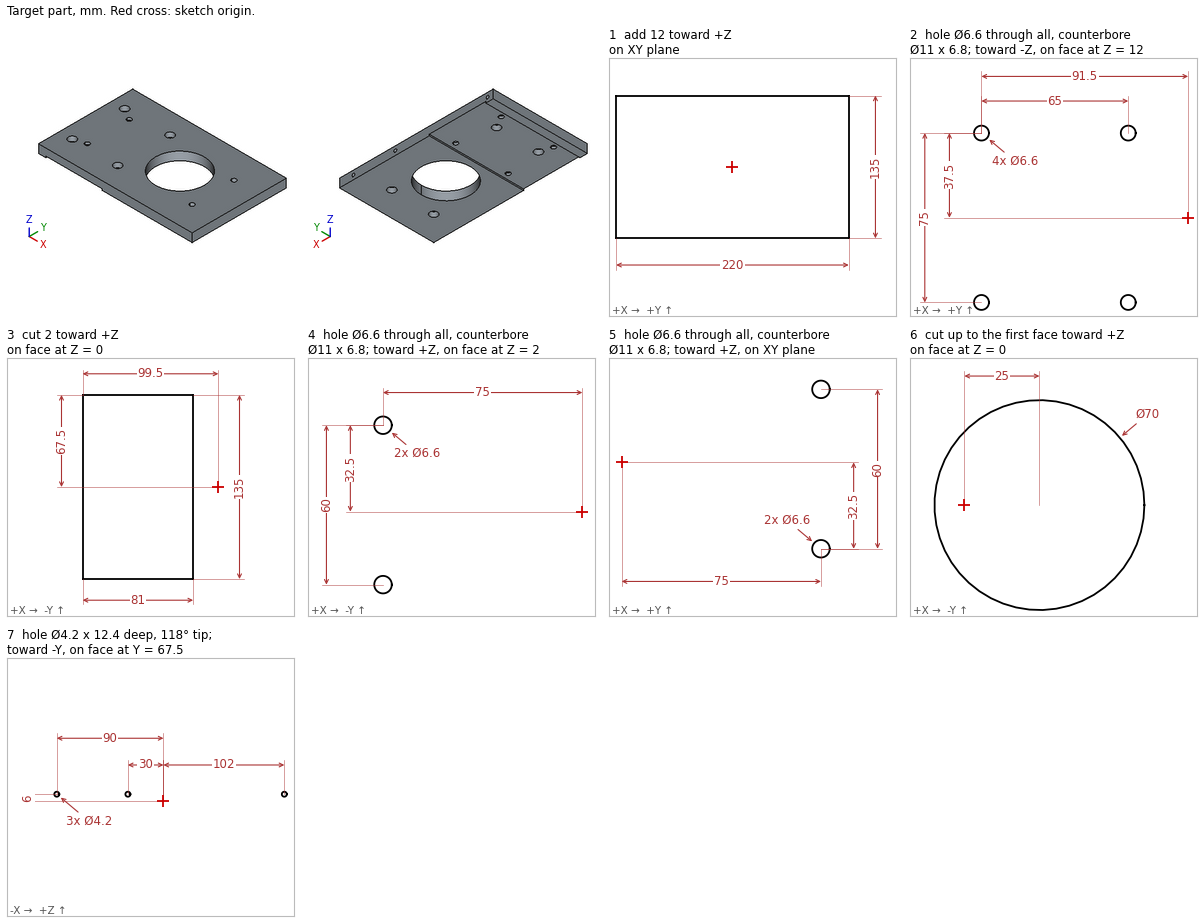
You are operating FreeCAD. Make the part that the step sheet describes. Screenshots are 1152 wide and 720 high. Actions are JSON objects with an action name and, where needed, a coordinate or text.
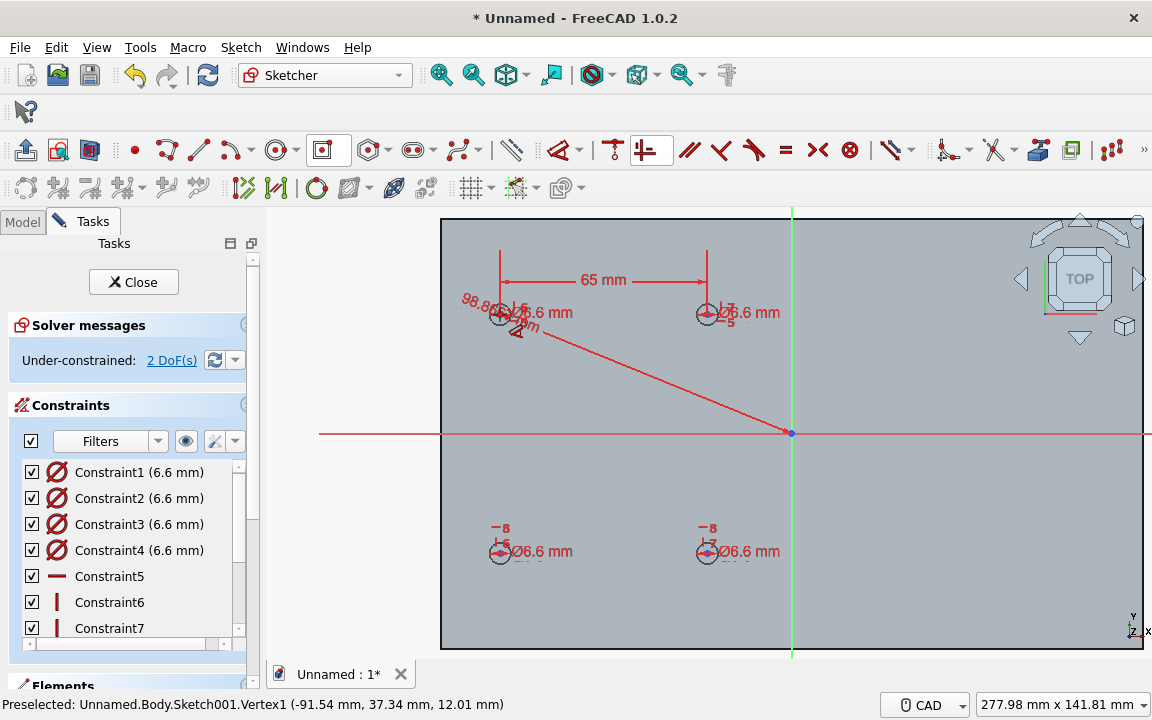
{"action": "left_click", "coordinate": [500, 554]}
{"action": "left_click", "coordinate": [466, 379]}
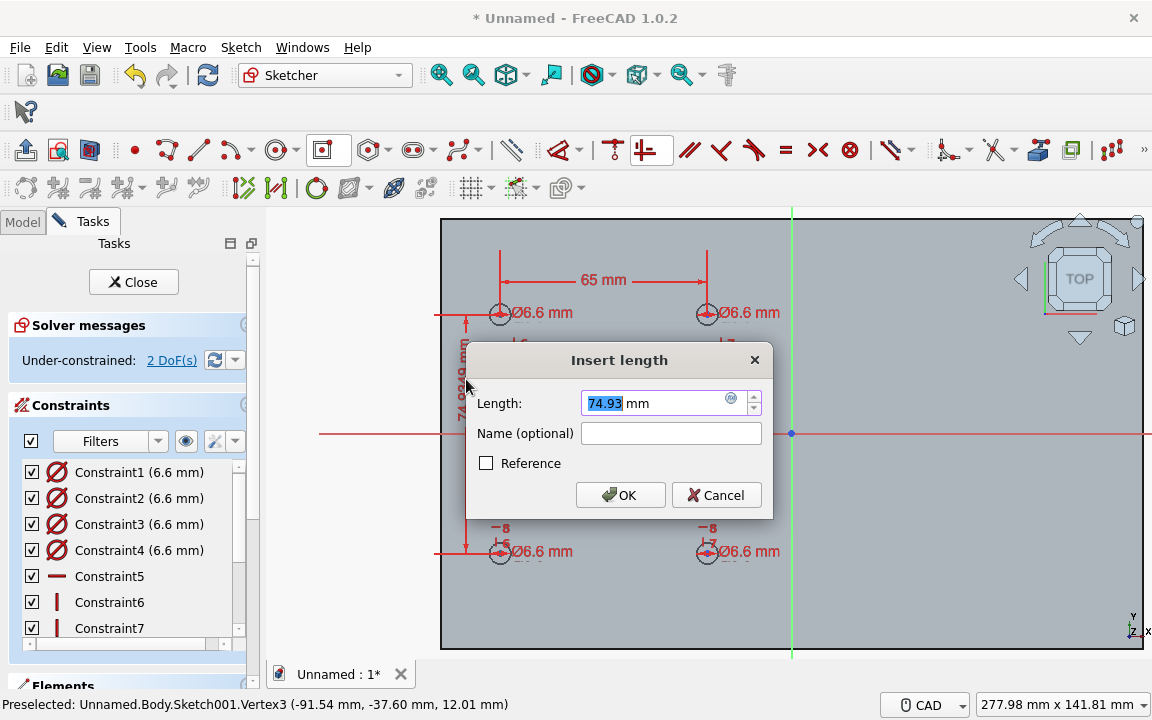
{"action": "type", "text": "75"}
{"action": "key", "text": "Return"}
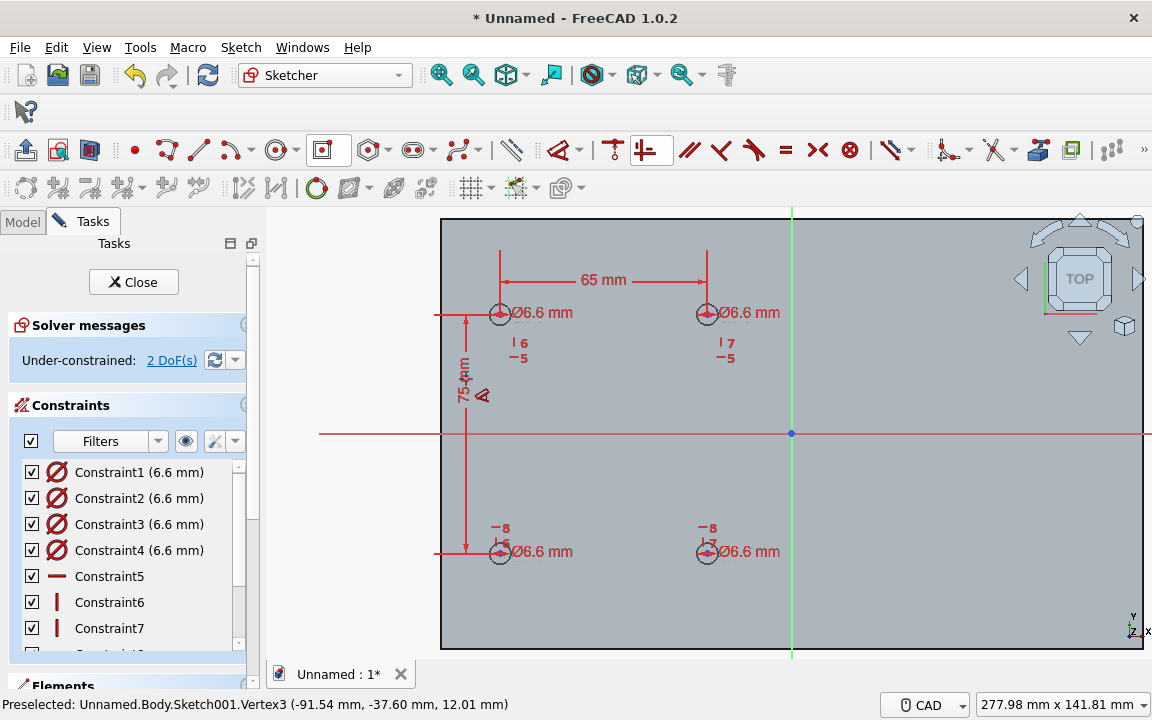
{"action": "left_click", "coordinate": [500, 315]}
{"action": "left_click", "coordinate": [713, 281]}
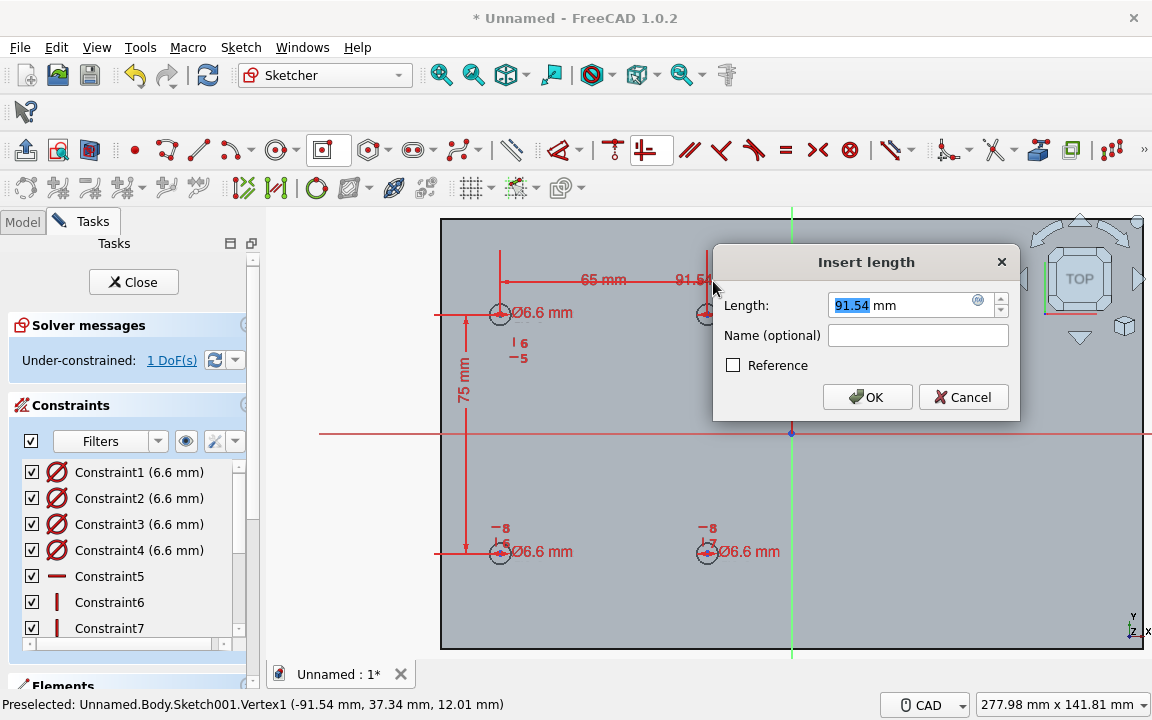
{"action": "type", "text": "91.5"}
{"action": "key", "text": "Return"}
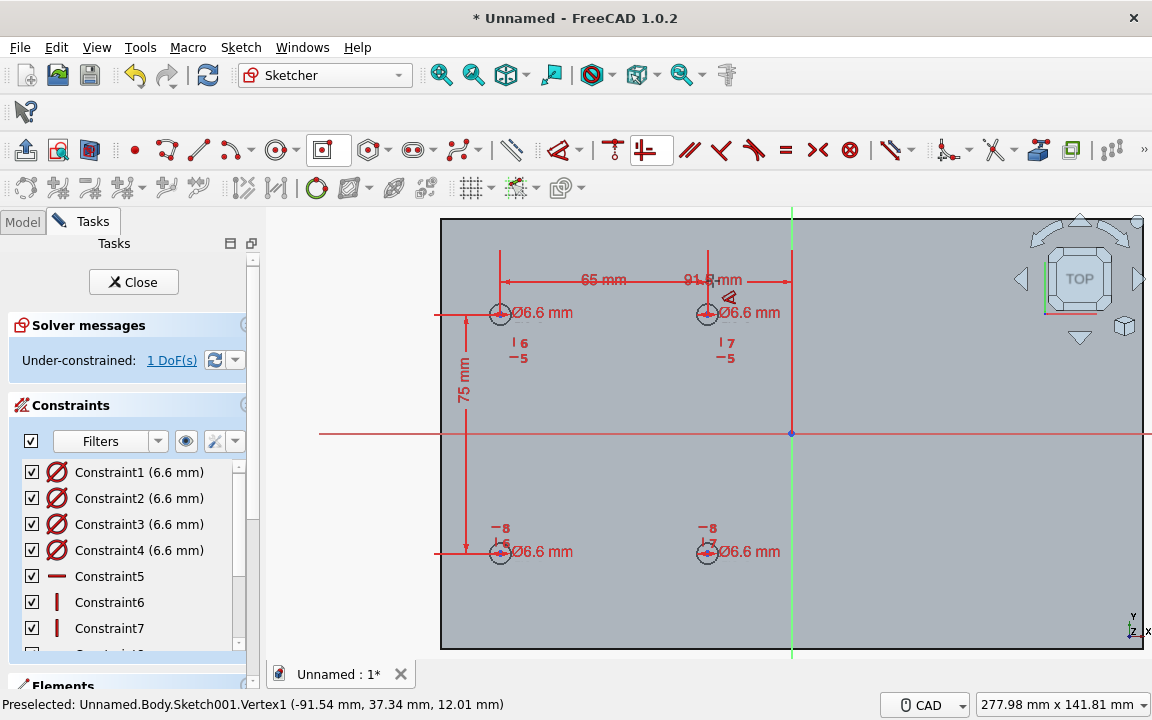
{"action": "left_click", "coordinate": [500, 315]}
{"action": "left_click", "coordinate": [826, 374]}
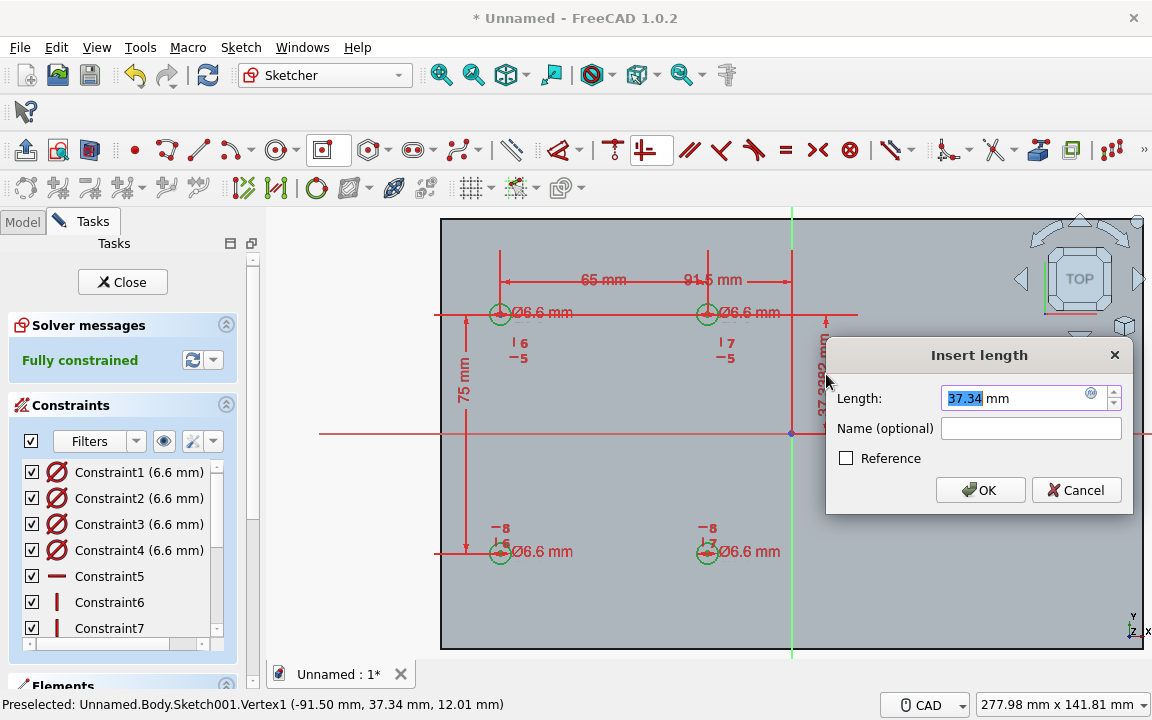
{"action": "type", "text": "37.5"}
{"action": "key", "text": "Return"}
{"action": "key", "text": "Escape"}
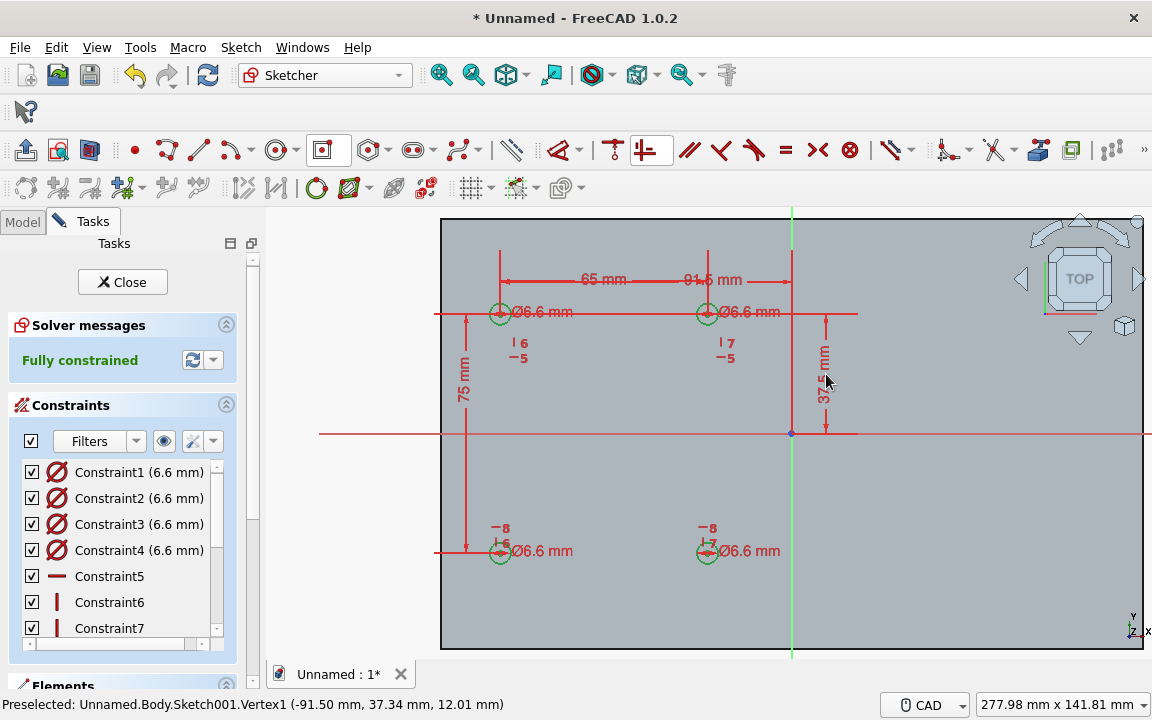
{"action": "left_click", "coordinate": [123, 282]}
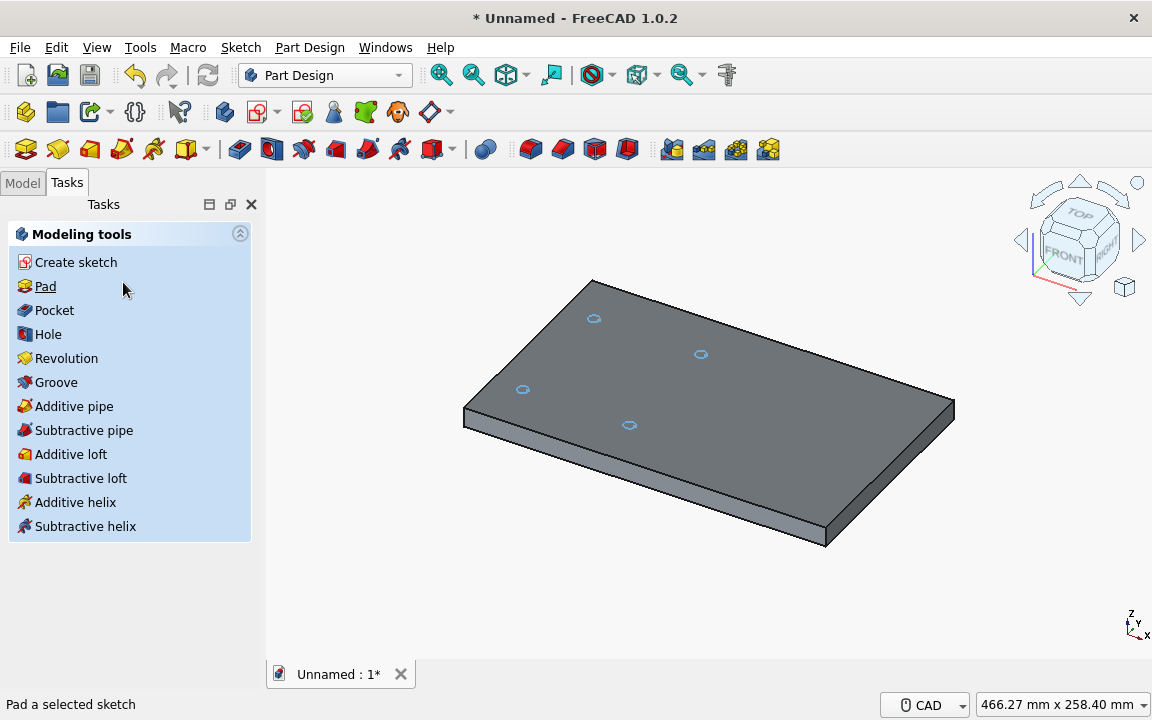
{"action": "left_click", "coordinate": [272, 150]}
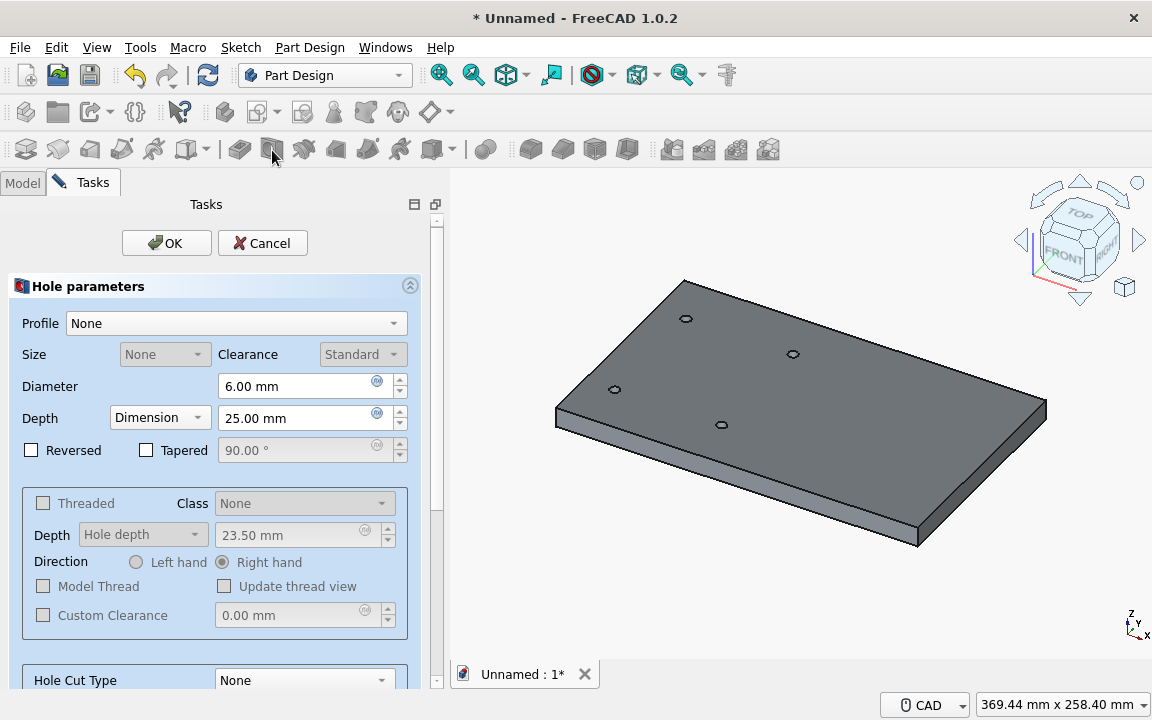
{"action": "triple_click", "coordinate": [305, 386]}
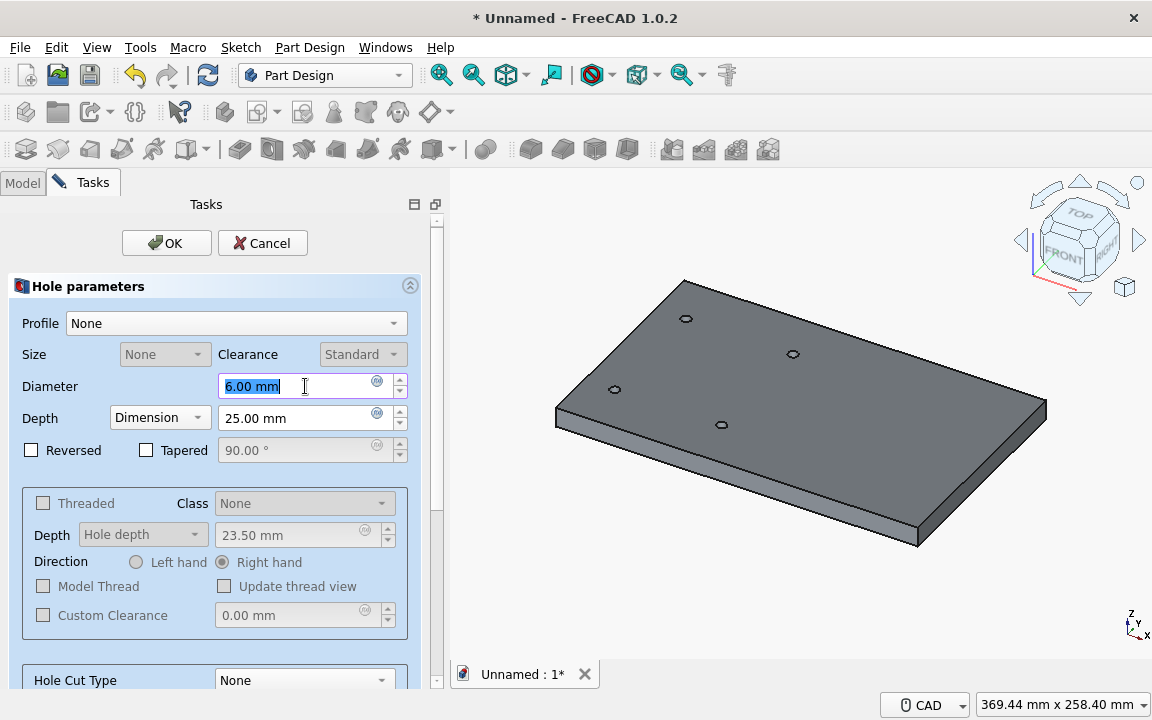
{"action": "type", "text": "6.6"}
{"action": "key", "text": "Tab"}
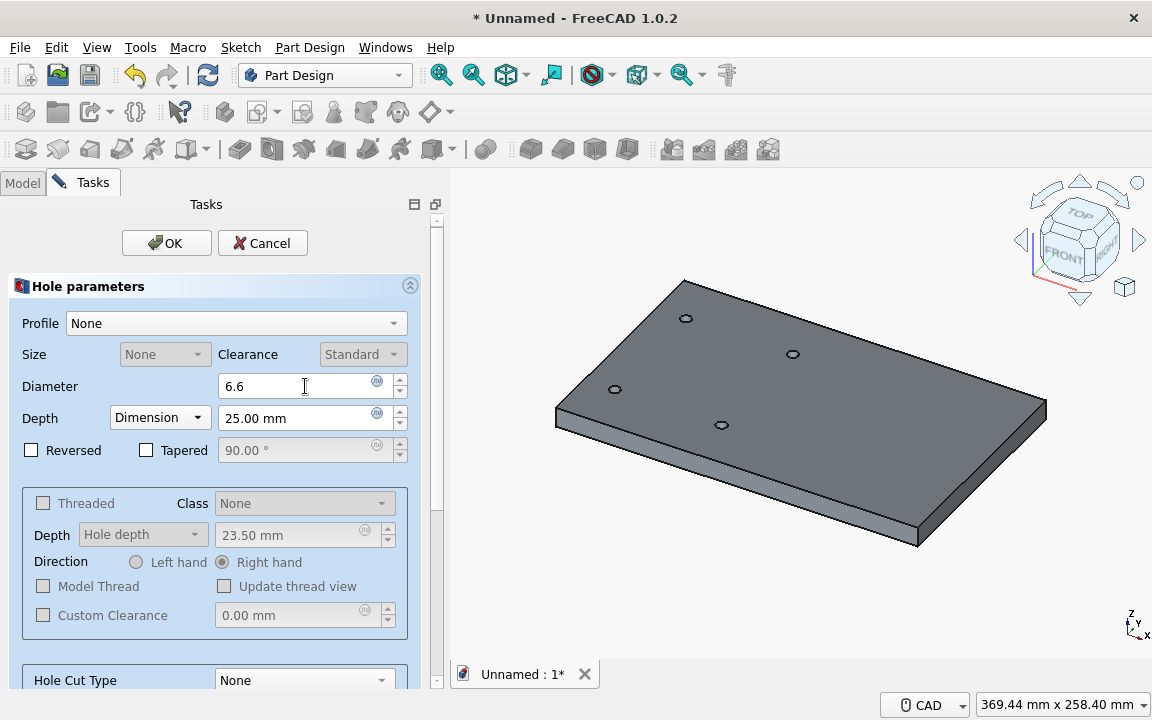
{"action": "left_click", "coordinate": [161, 418]}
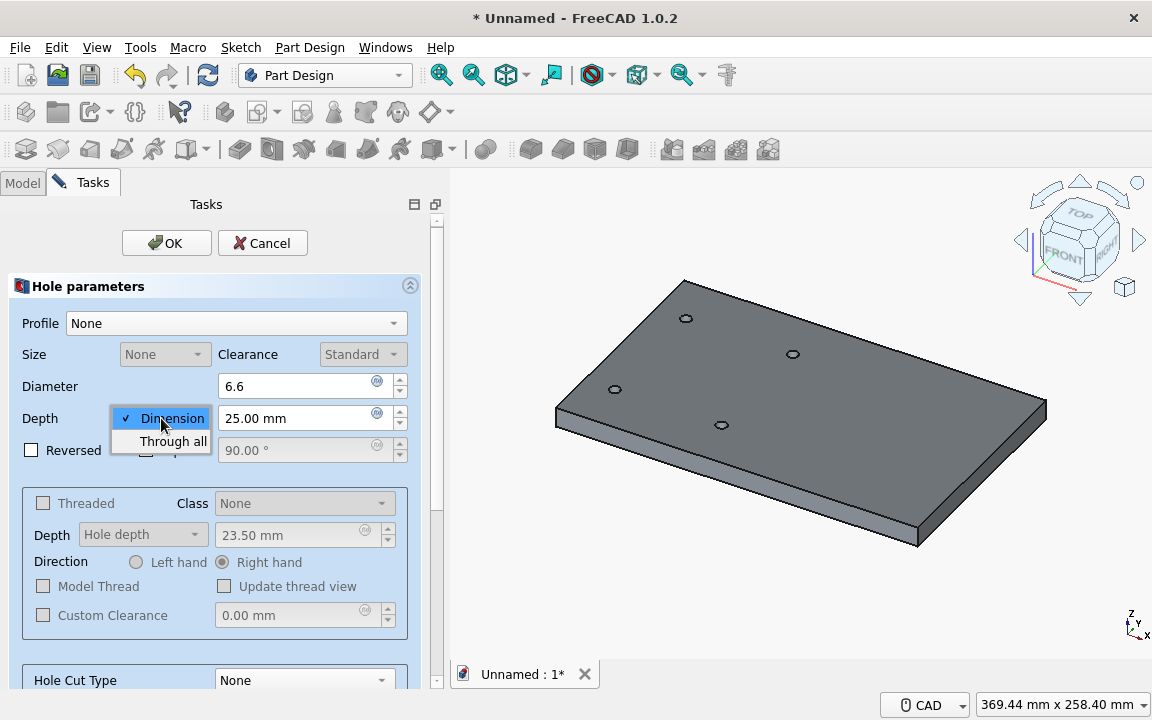
{"action": "left_click", "coordinate": [160, 442]}